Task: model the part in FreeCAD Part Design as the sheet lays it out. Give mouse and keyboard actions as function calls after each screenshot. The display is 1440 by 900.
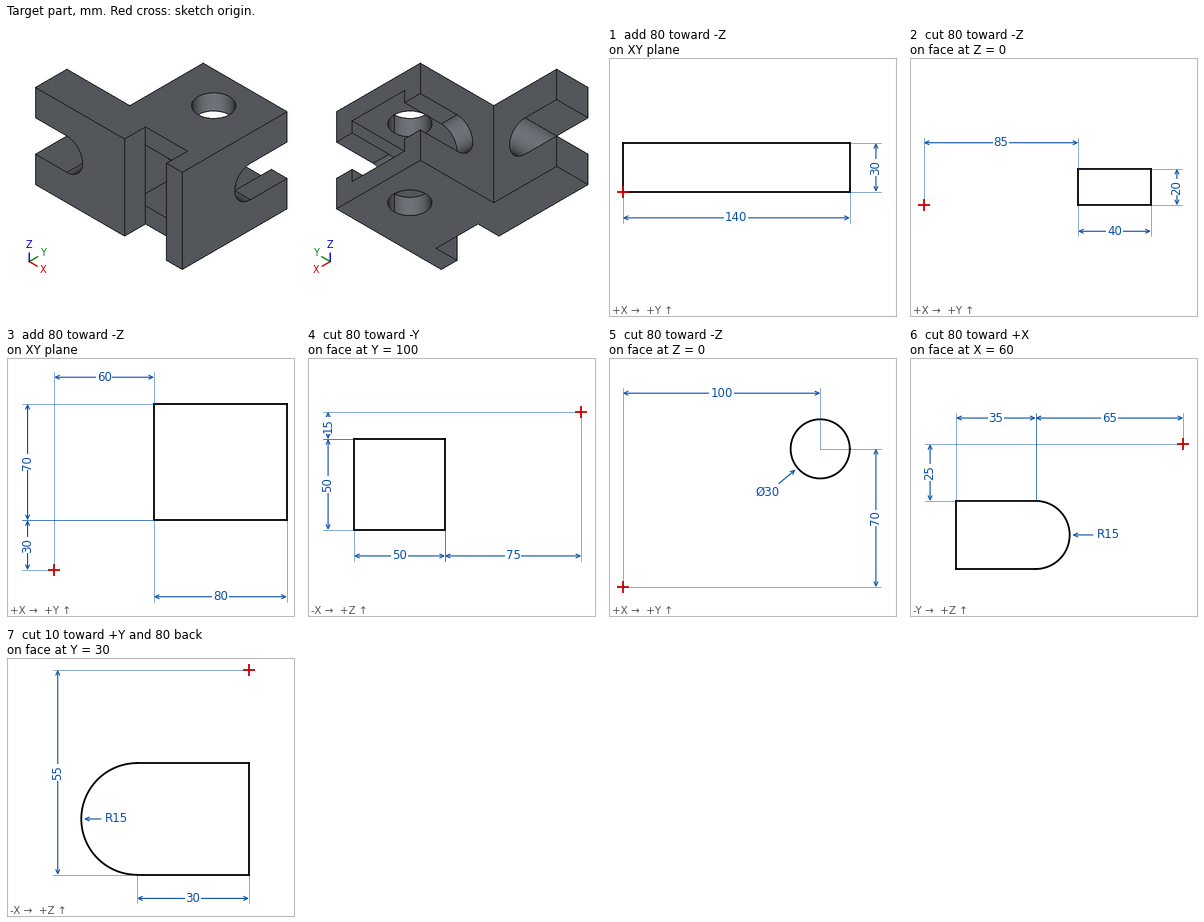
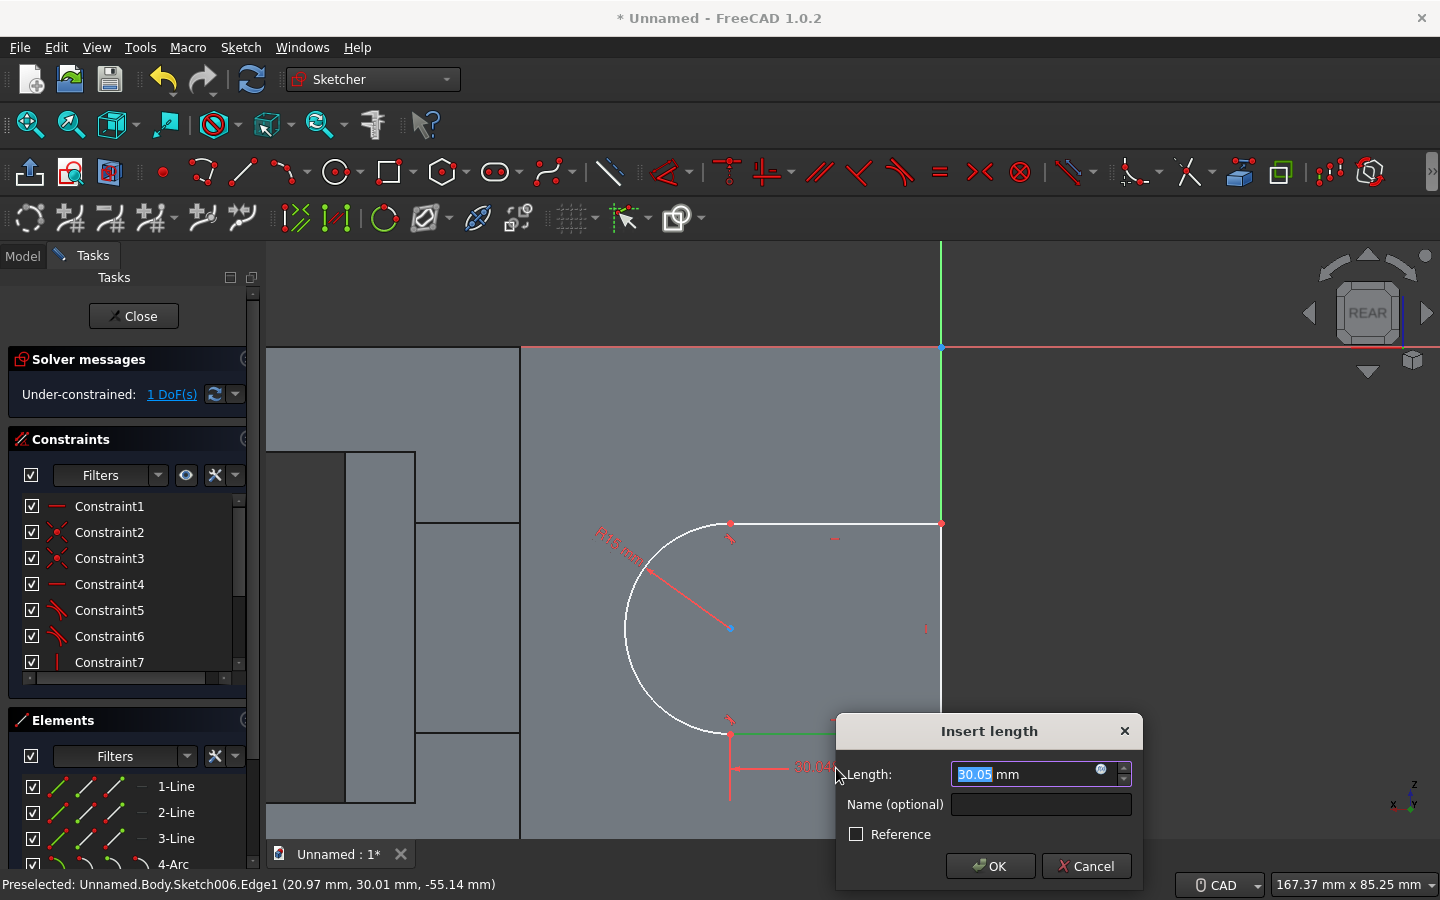
text(30)
key(Return)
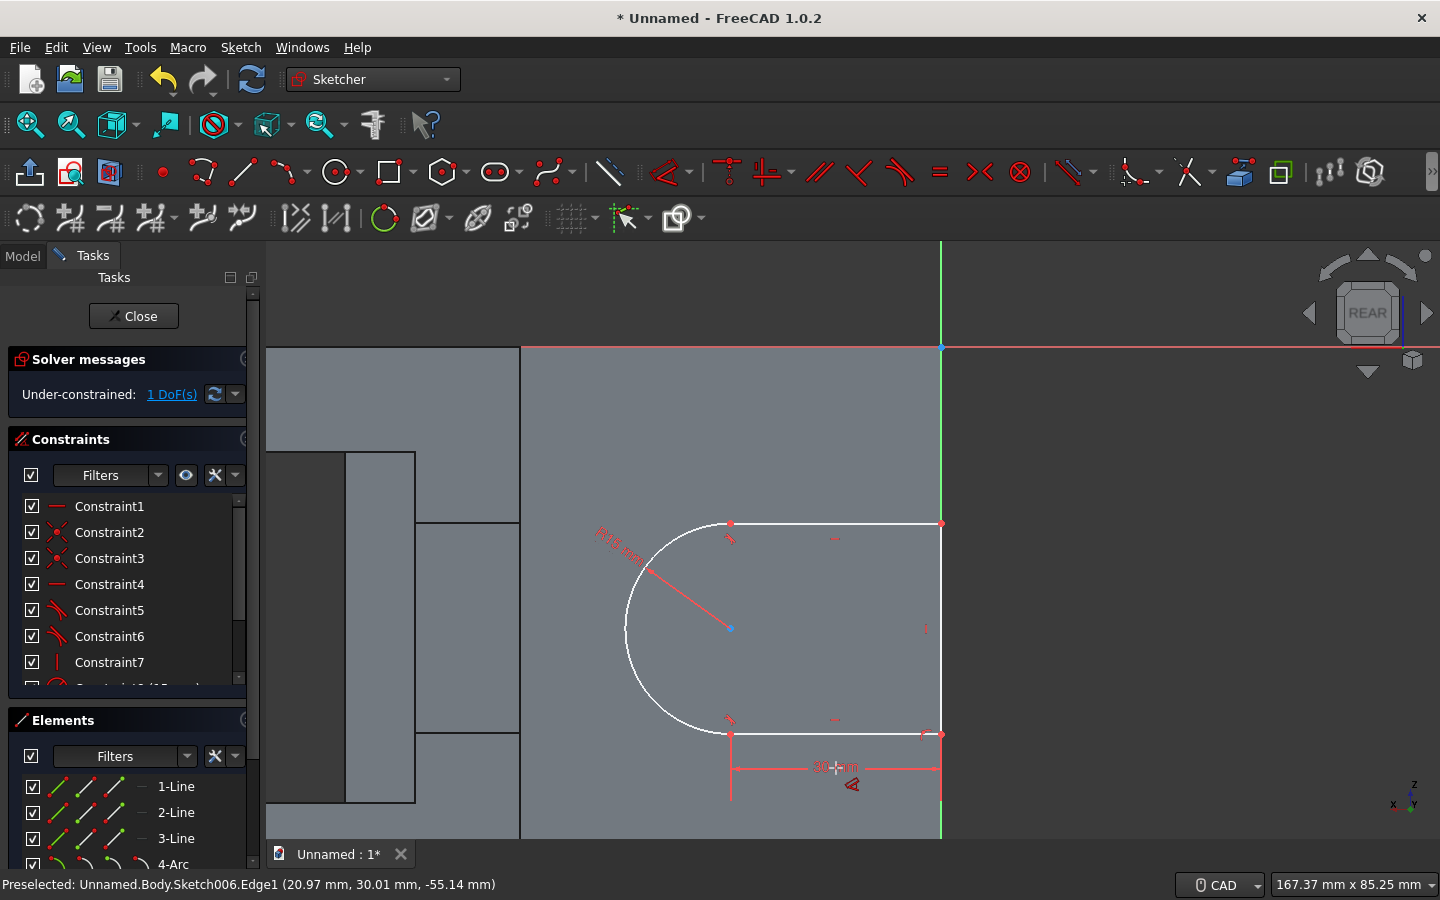
click(731, 734)
click(975, 541)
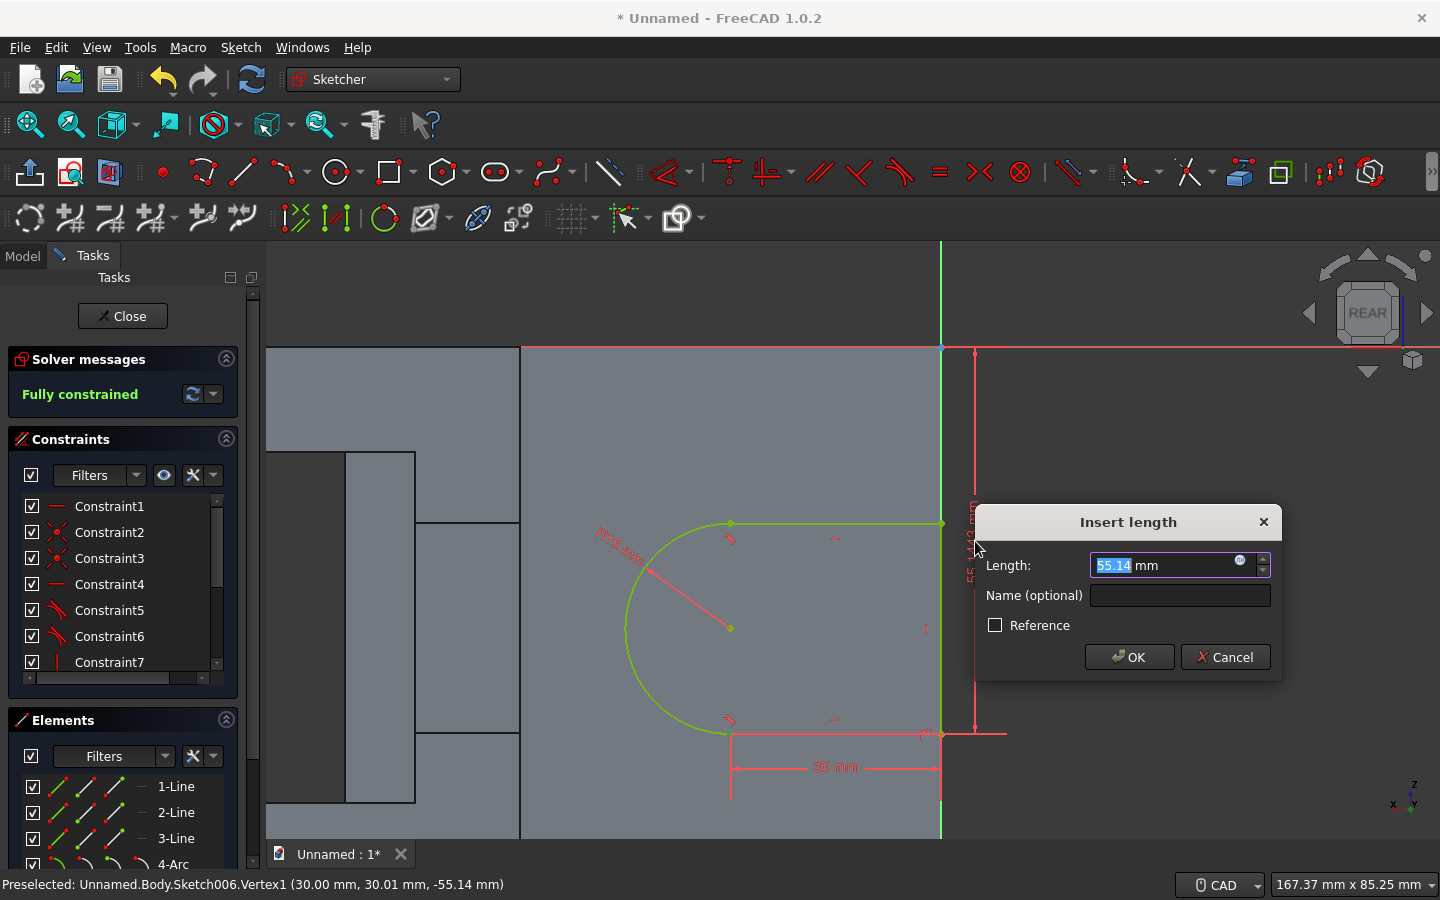
text(55)
key(Return)
key(Escape)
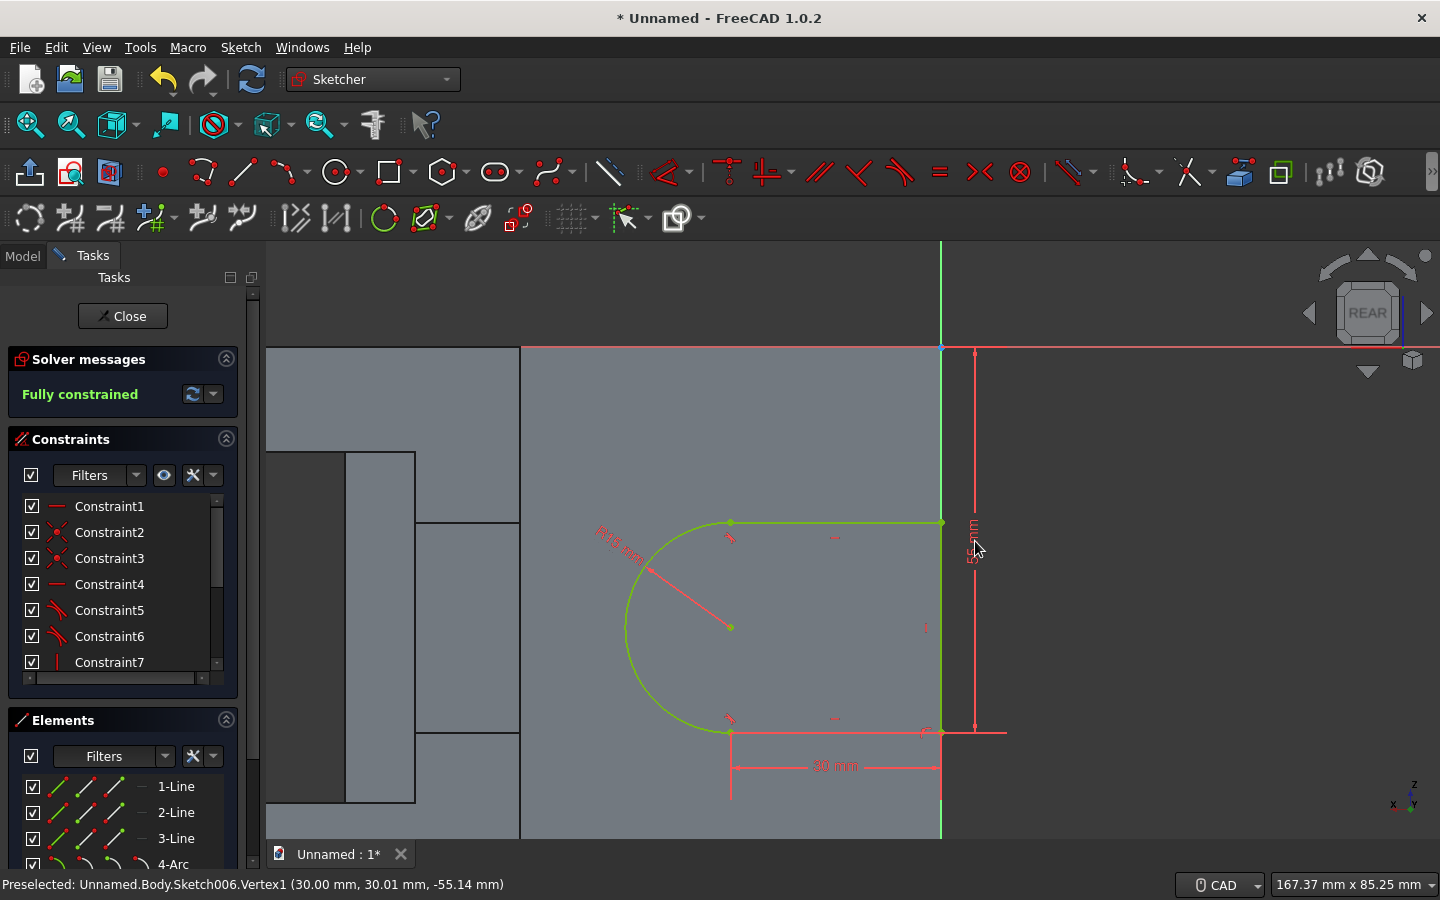
click(123, 316)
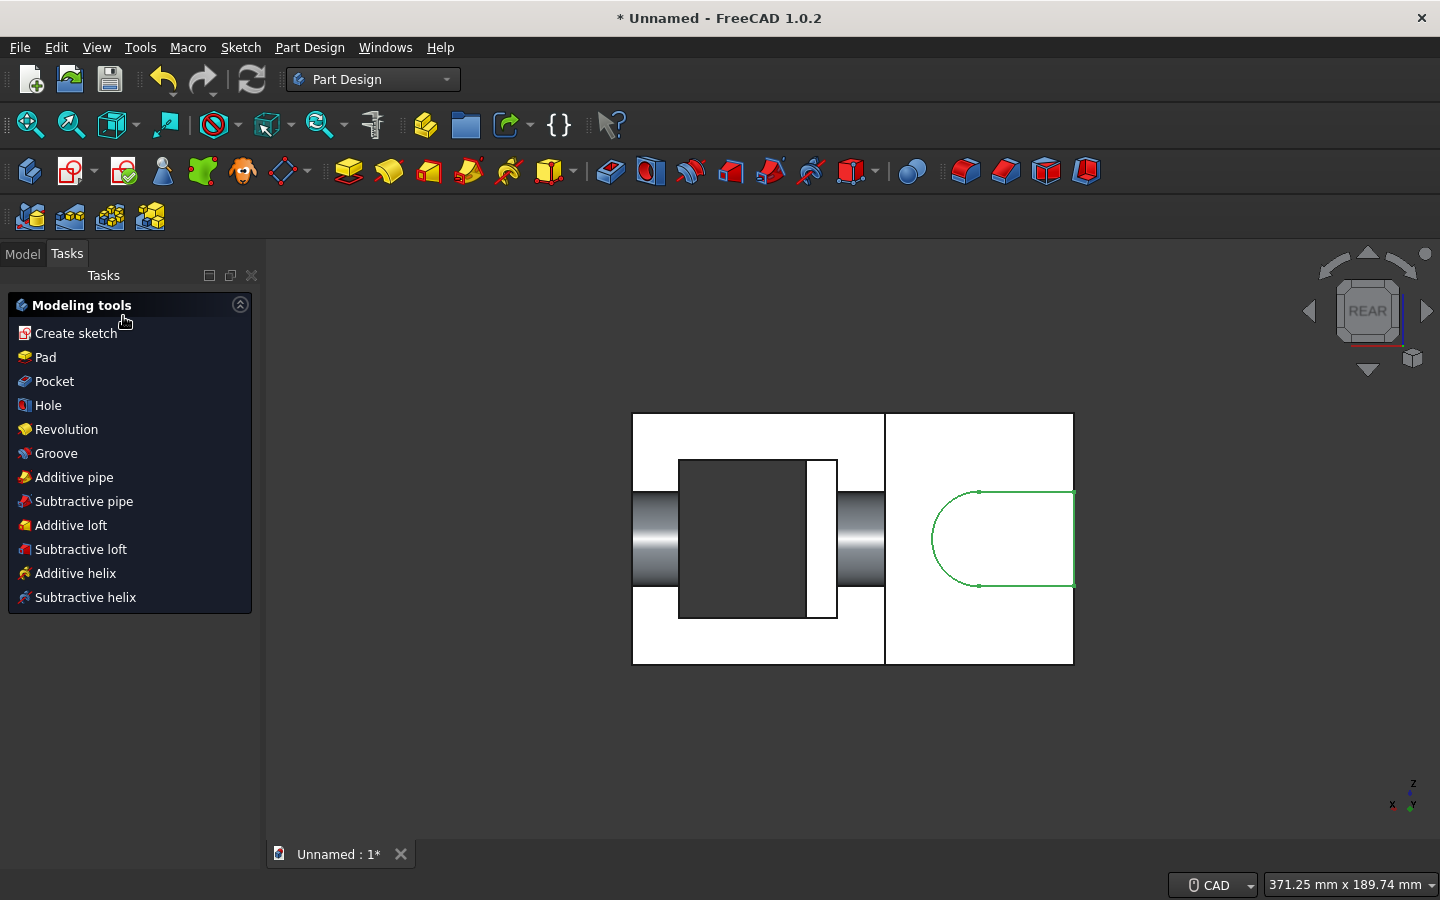
click(612, 172)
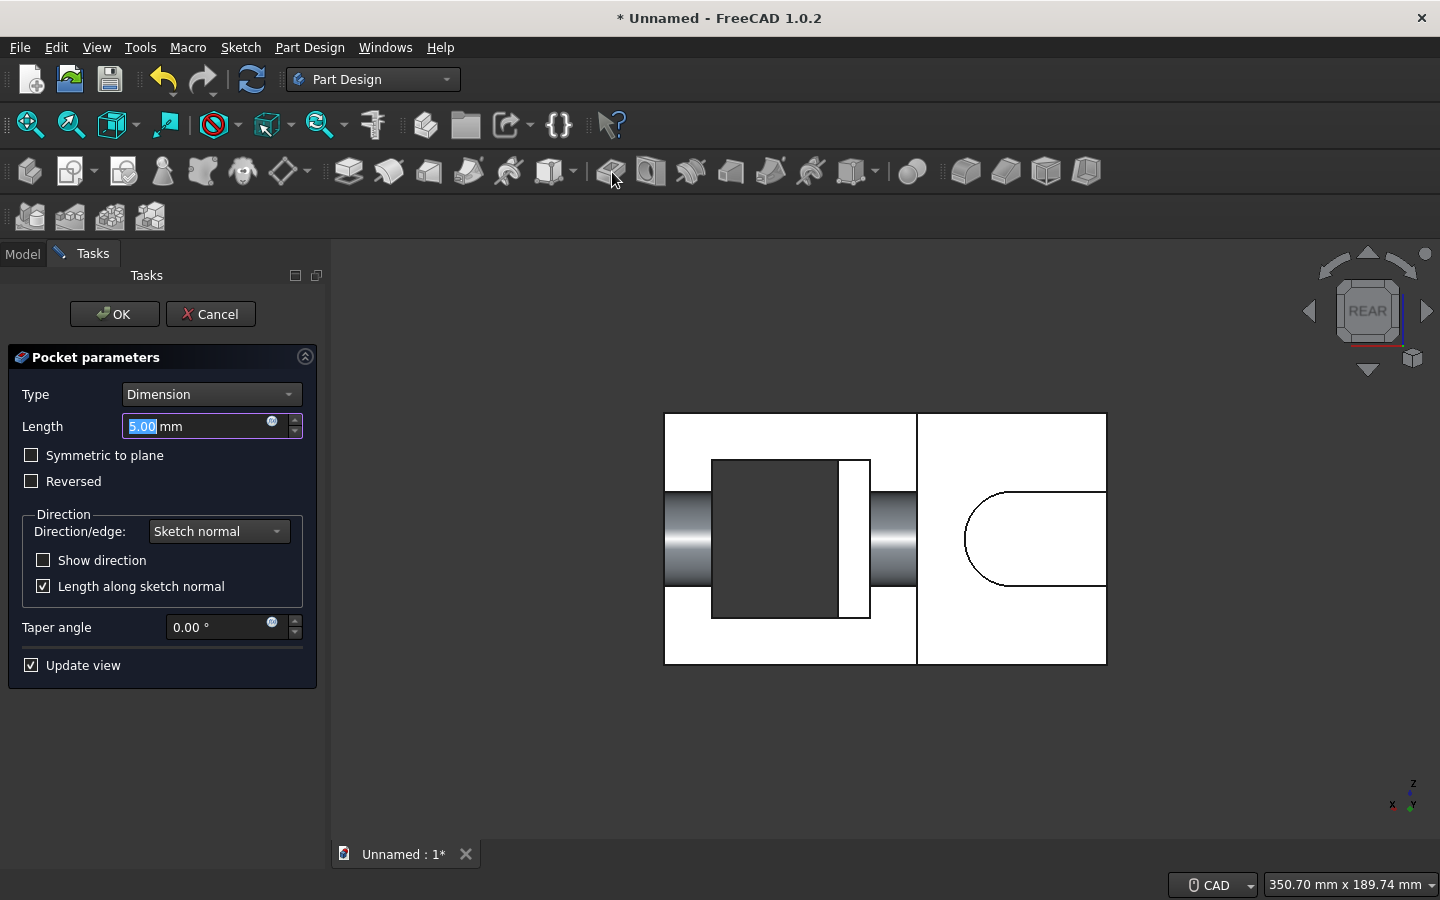
click(212, 394)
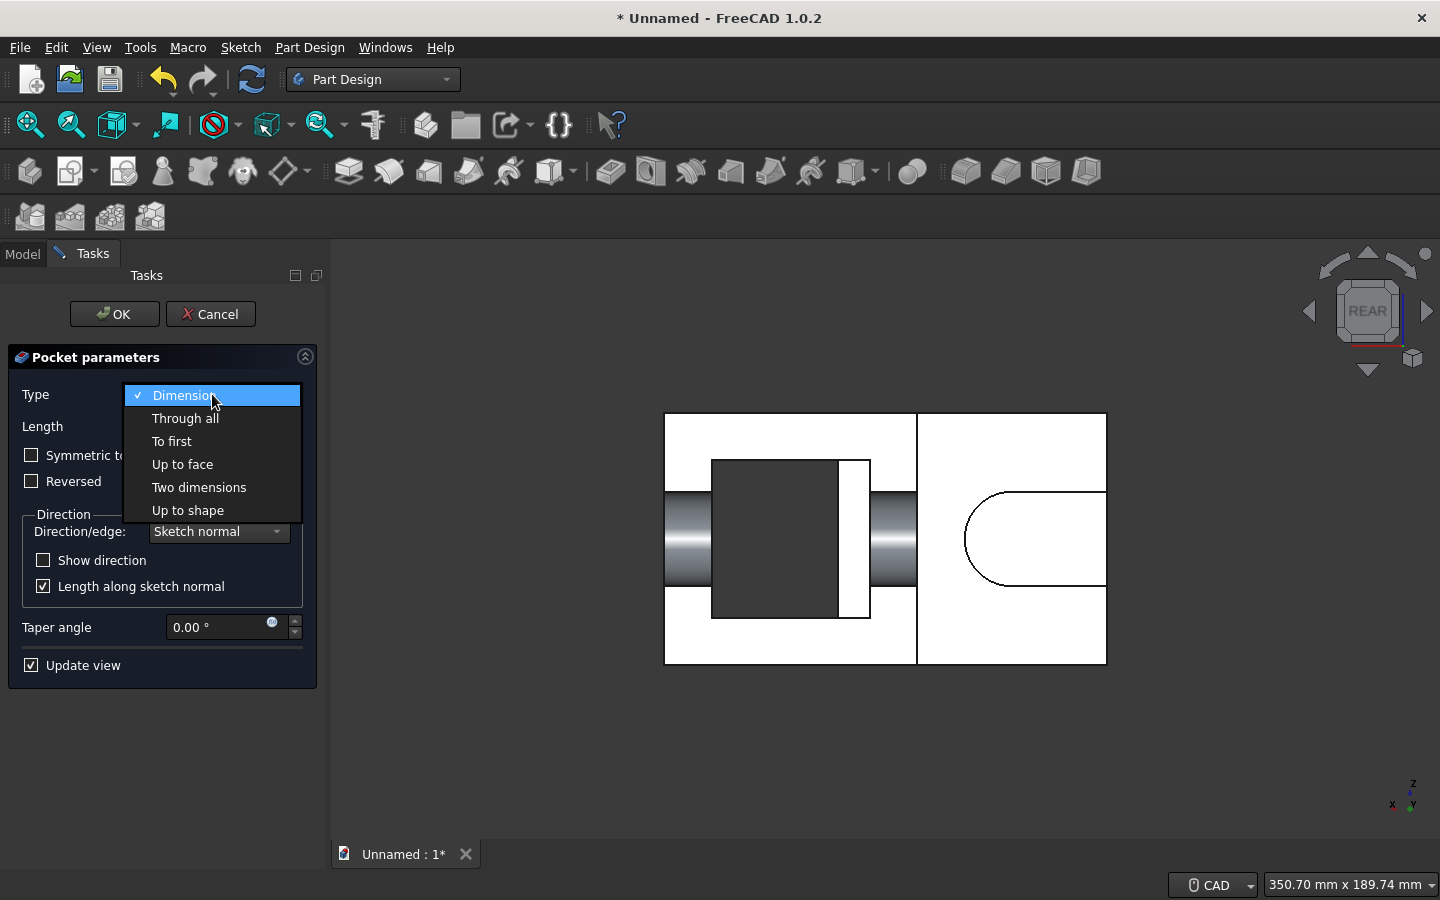
click(212, 488)